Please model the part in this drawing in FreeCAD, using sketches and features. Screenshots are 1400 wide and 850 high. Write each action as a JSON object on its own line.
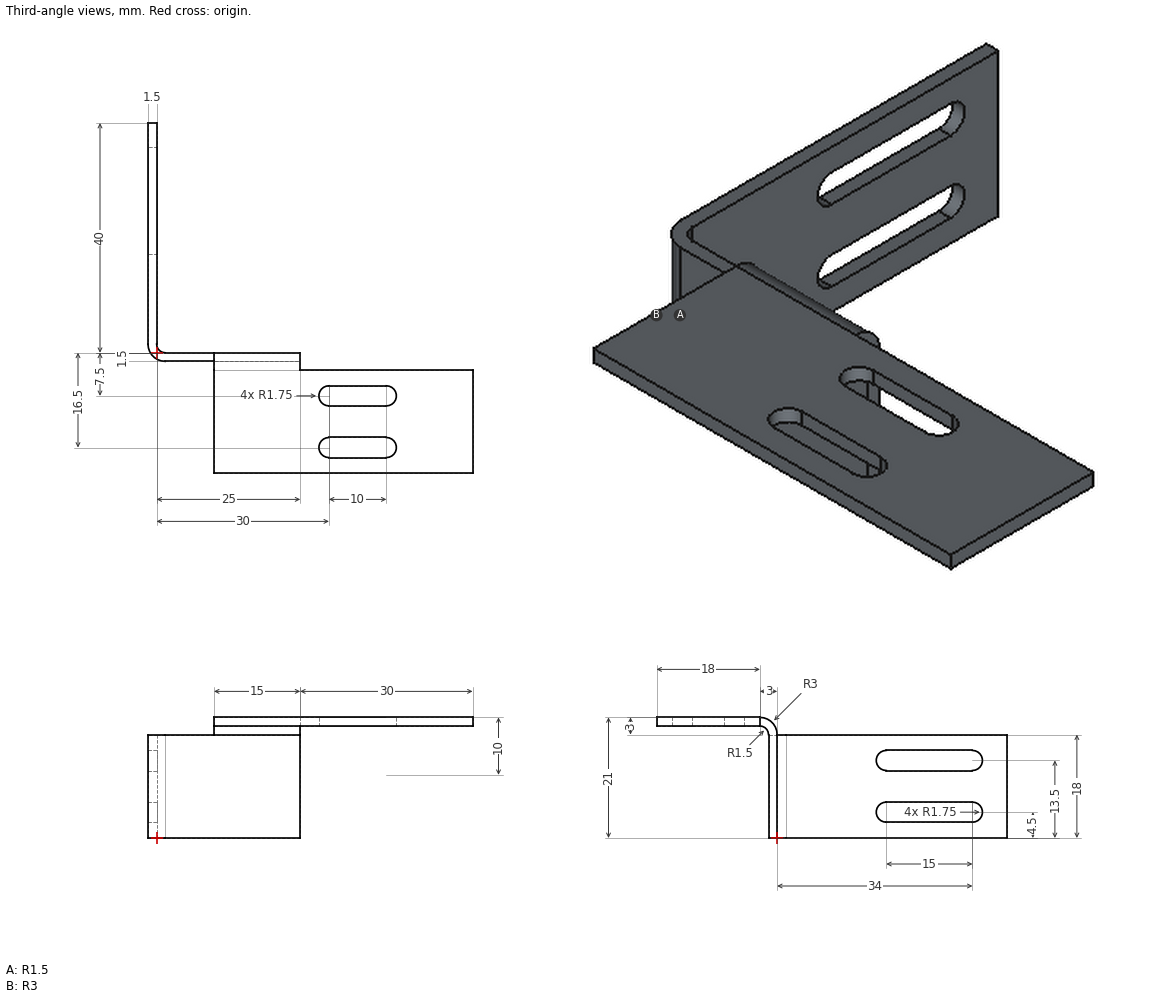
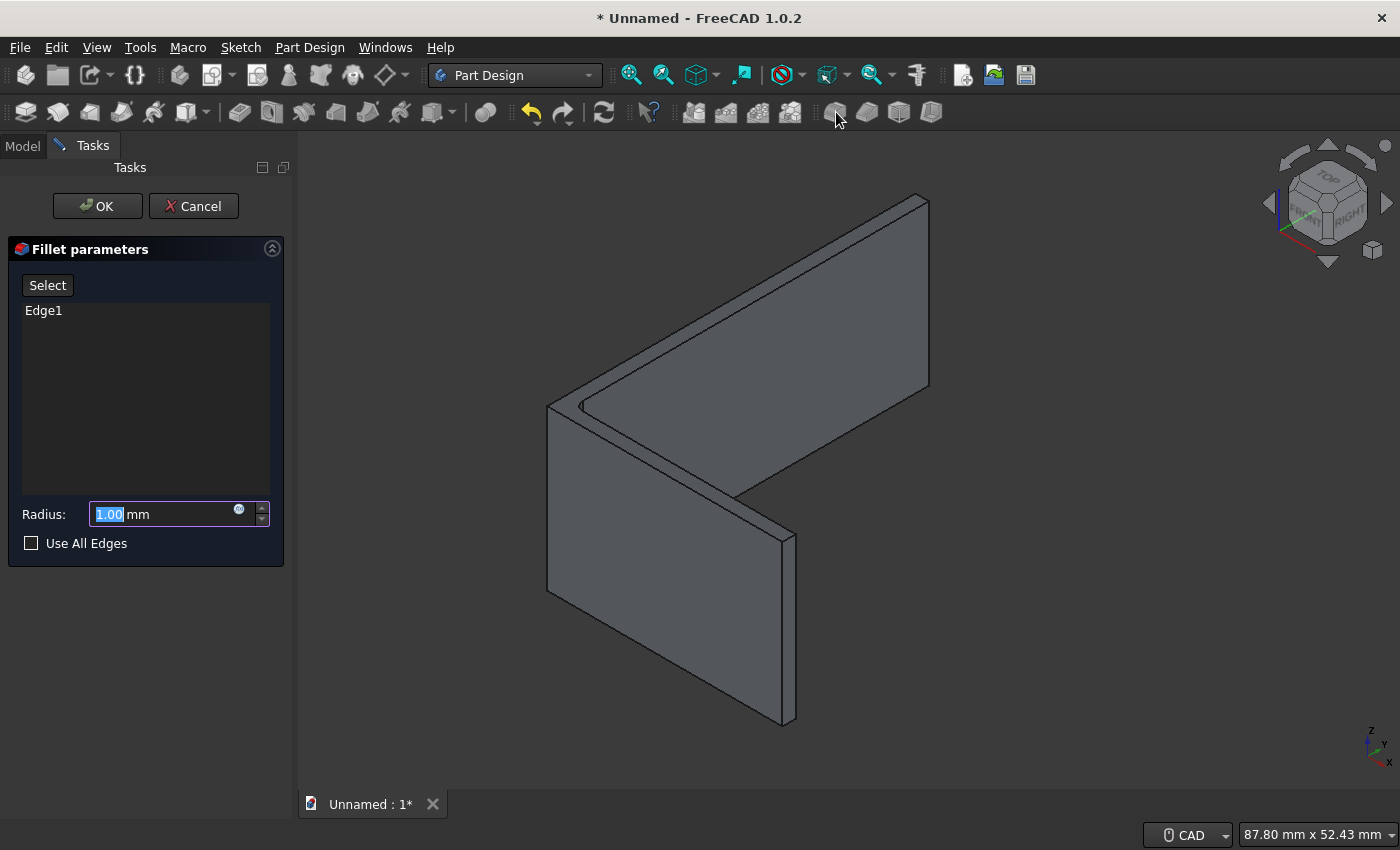
{"action": "type", "text": "1.5"}
{"action": "key", "text": "Tab"}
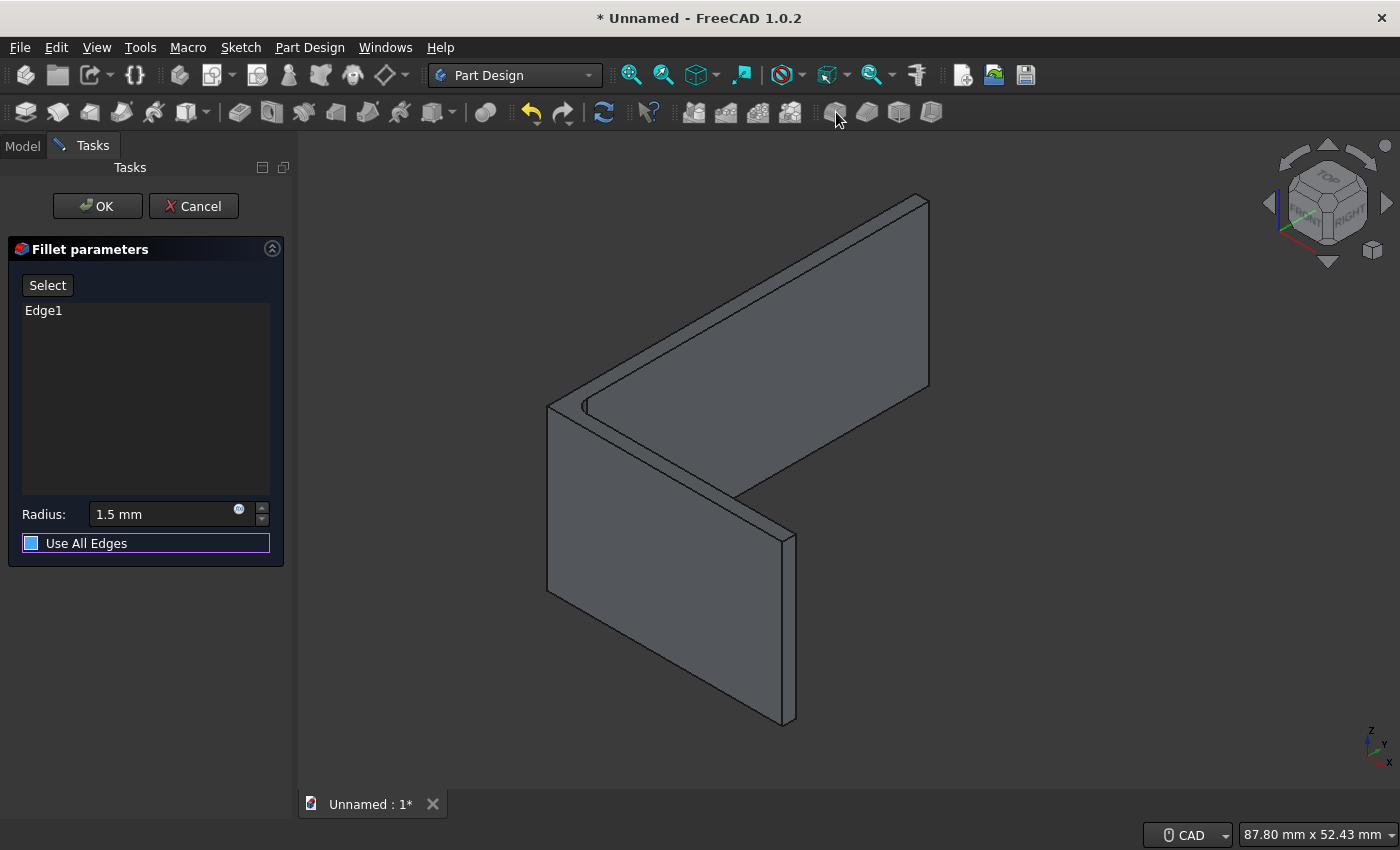
{"action": "left_click", "coordinate": [98, 206]}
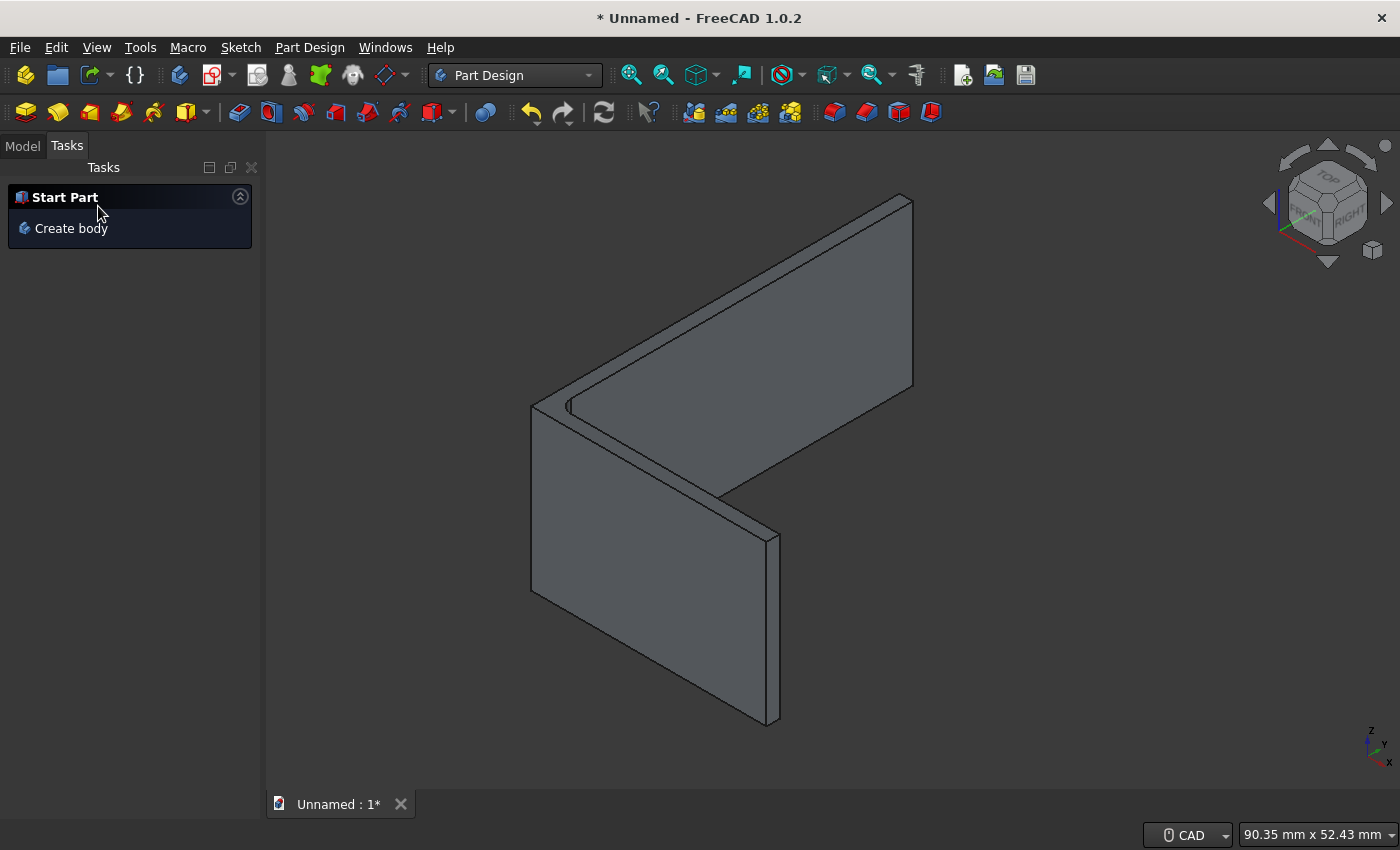
{"action": "key", "text": "2"}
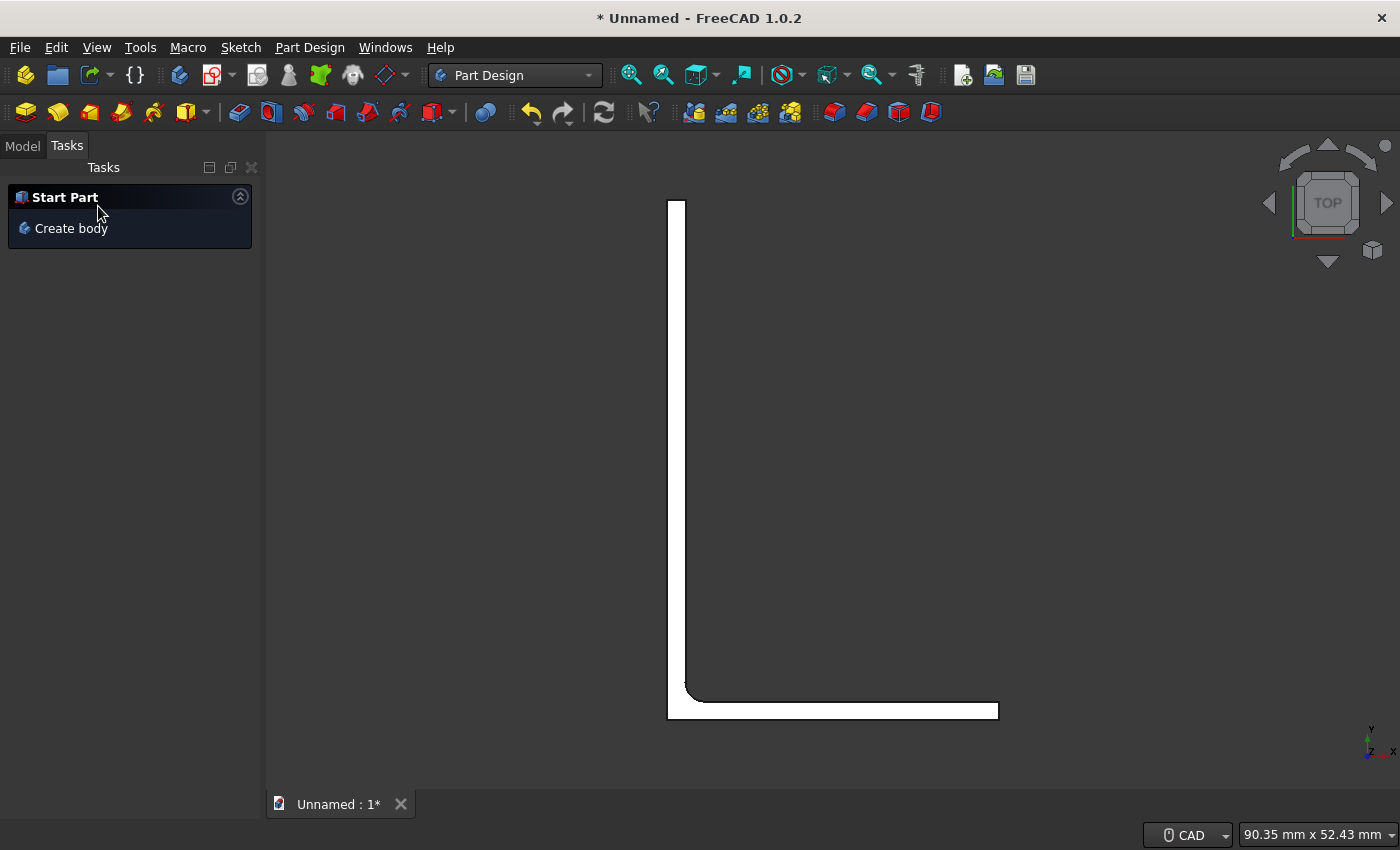
{"action": "key", "text": "0"}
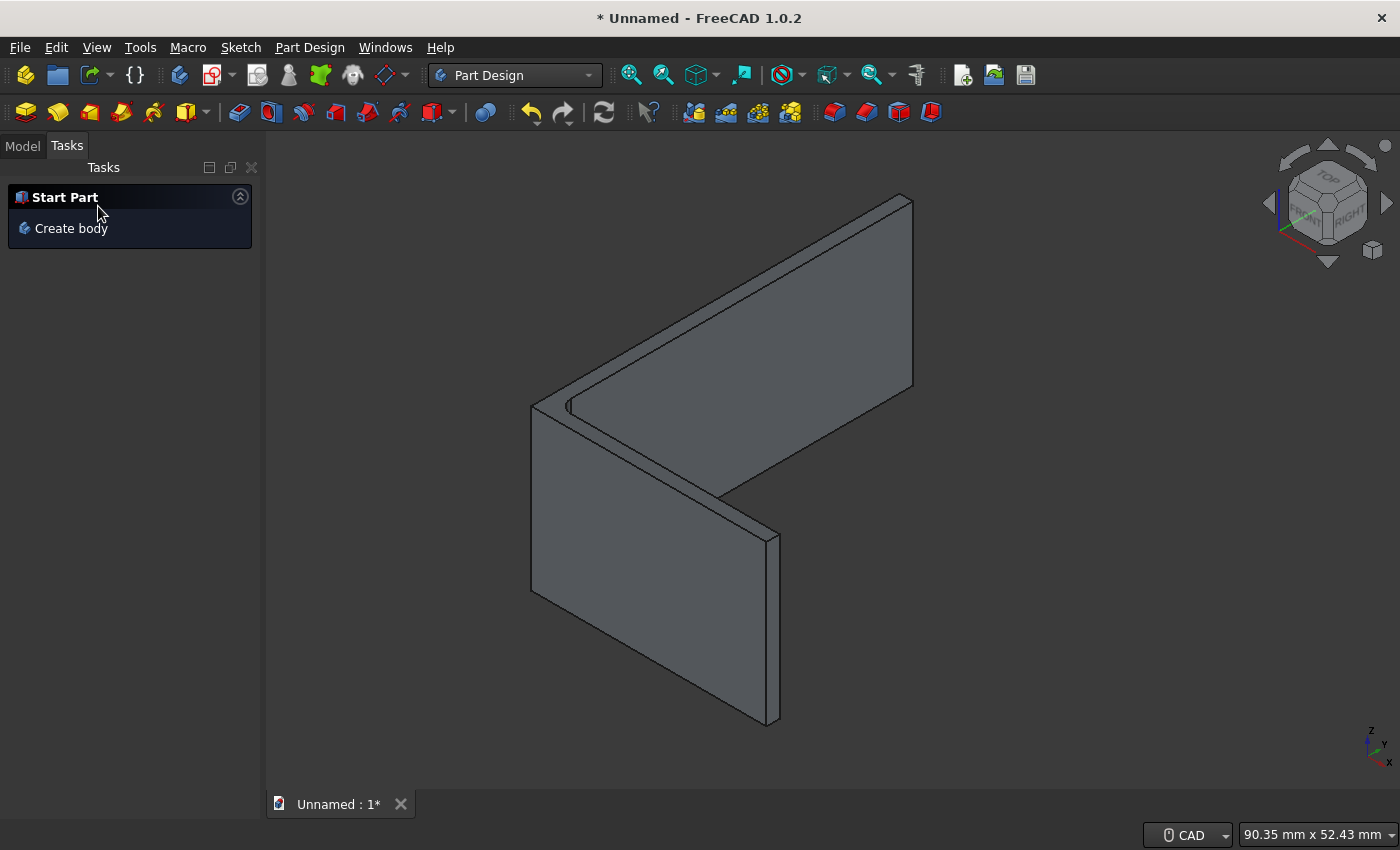
{"action": "key", "text": "1"}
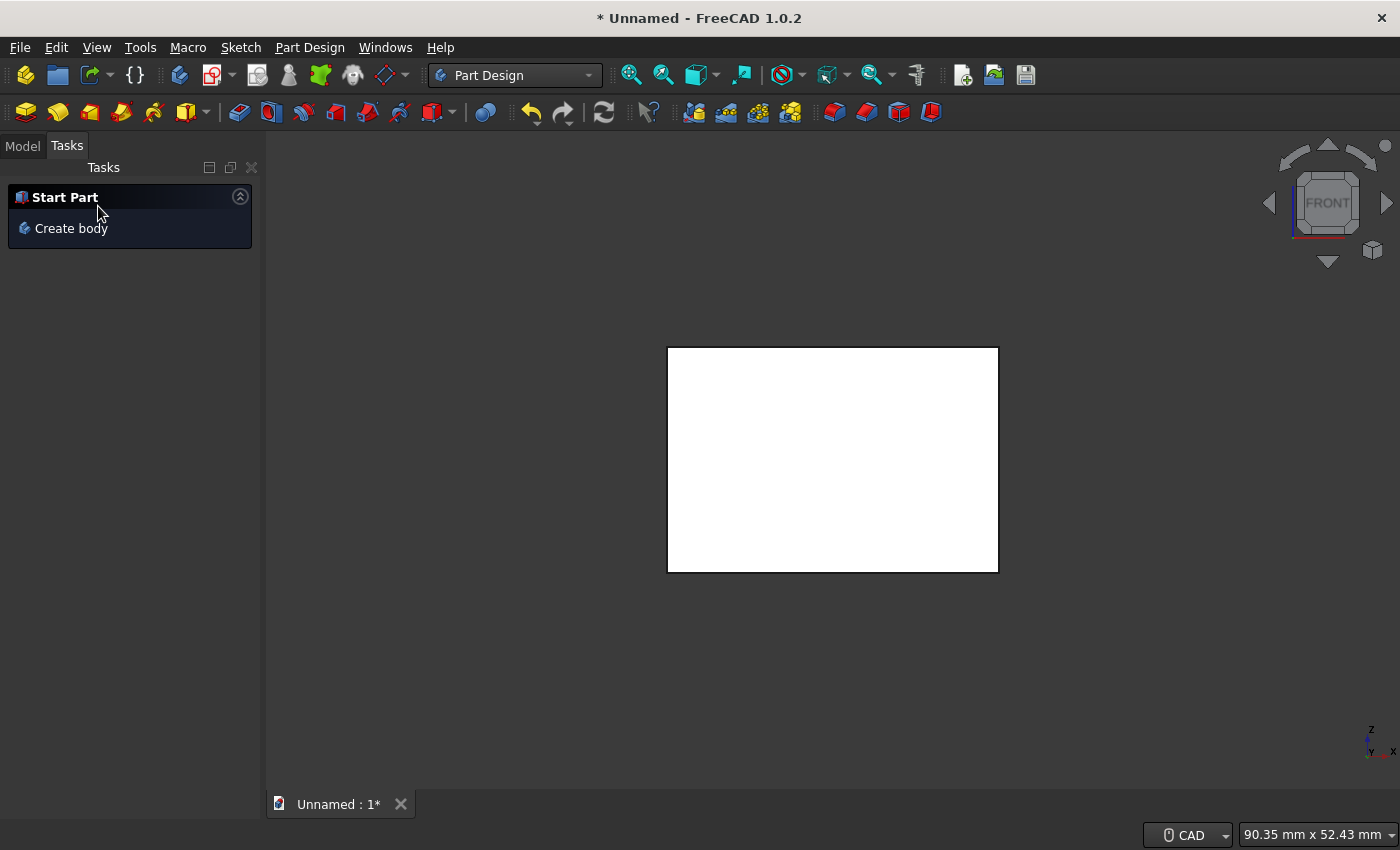
{"action": "left_click", "coordinate": [632, 76]}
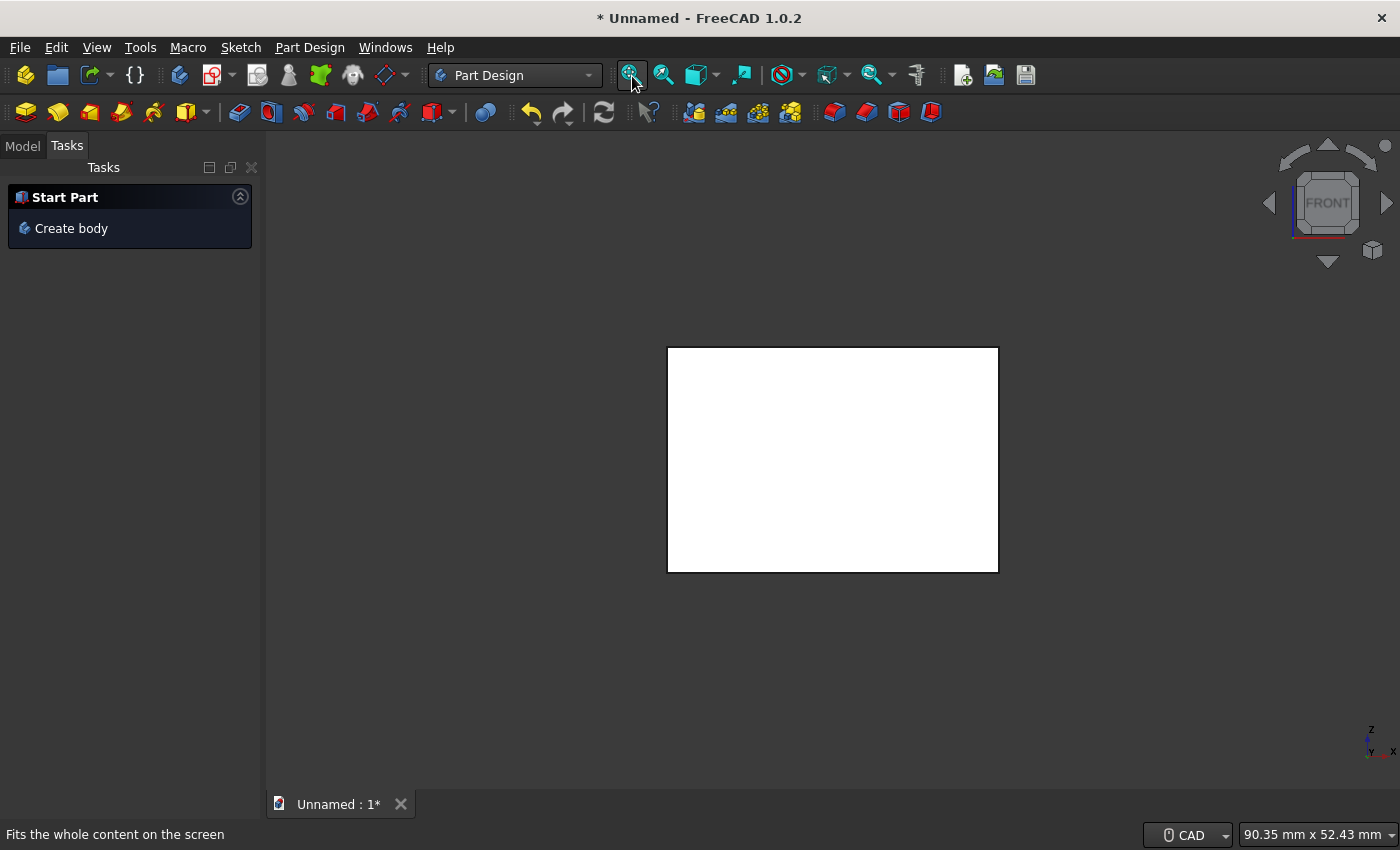
{"action": "left_click", "coordinate": [667, 459]}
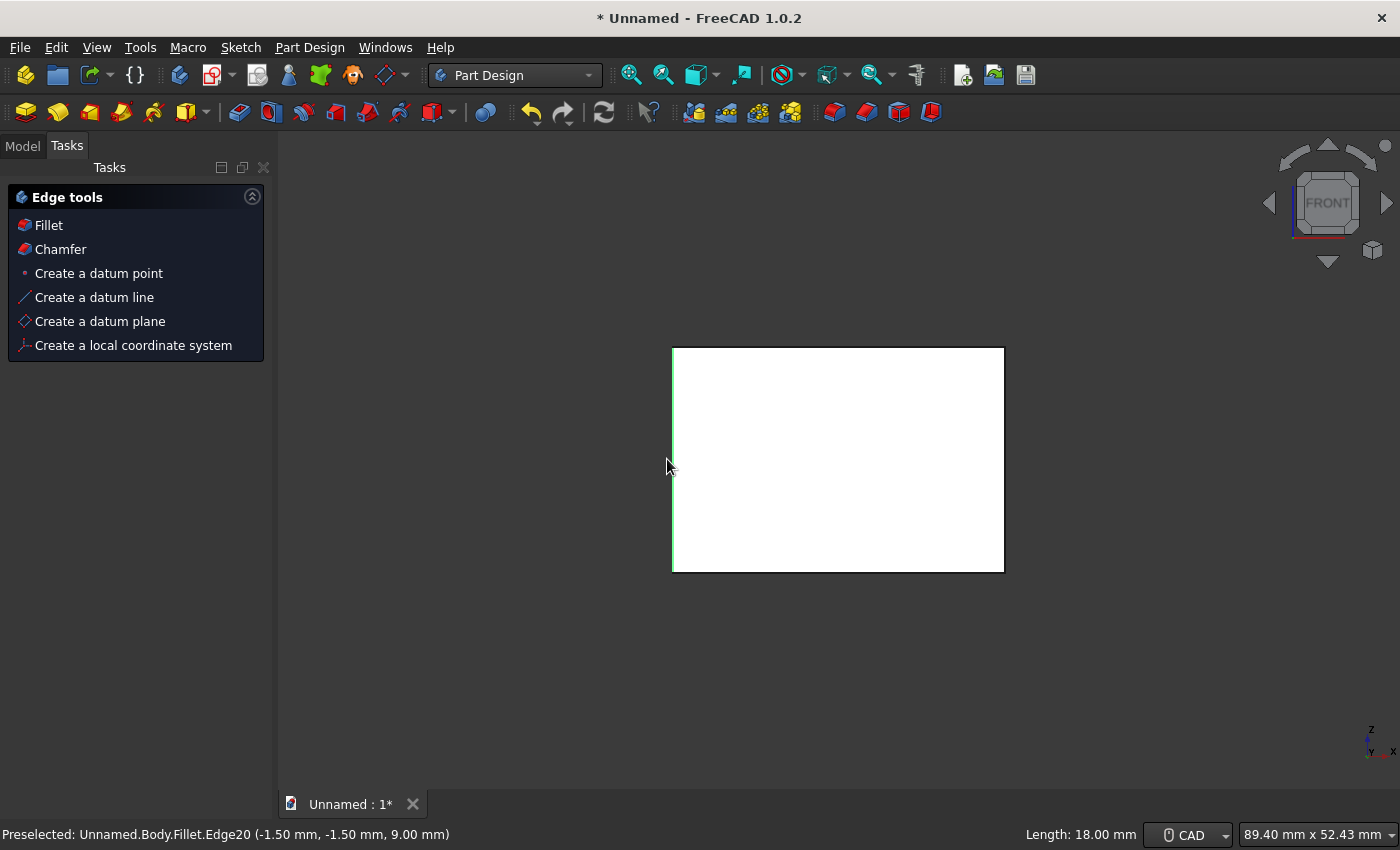
{"action": "left_click", "coordinate": [836, 112]}